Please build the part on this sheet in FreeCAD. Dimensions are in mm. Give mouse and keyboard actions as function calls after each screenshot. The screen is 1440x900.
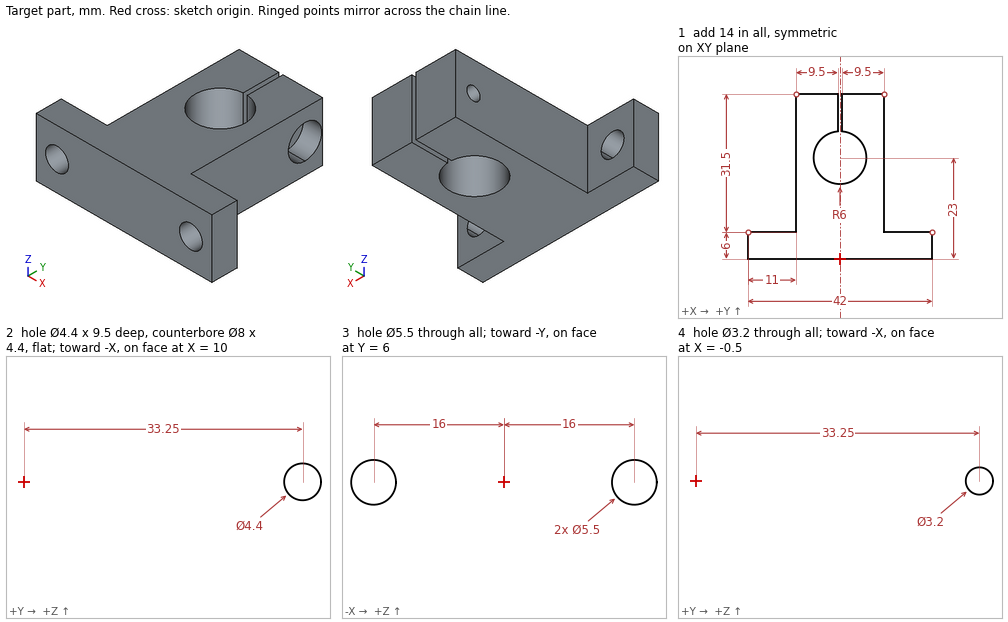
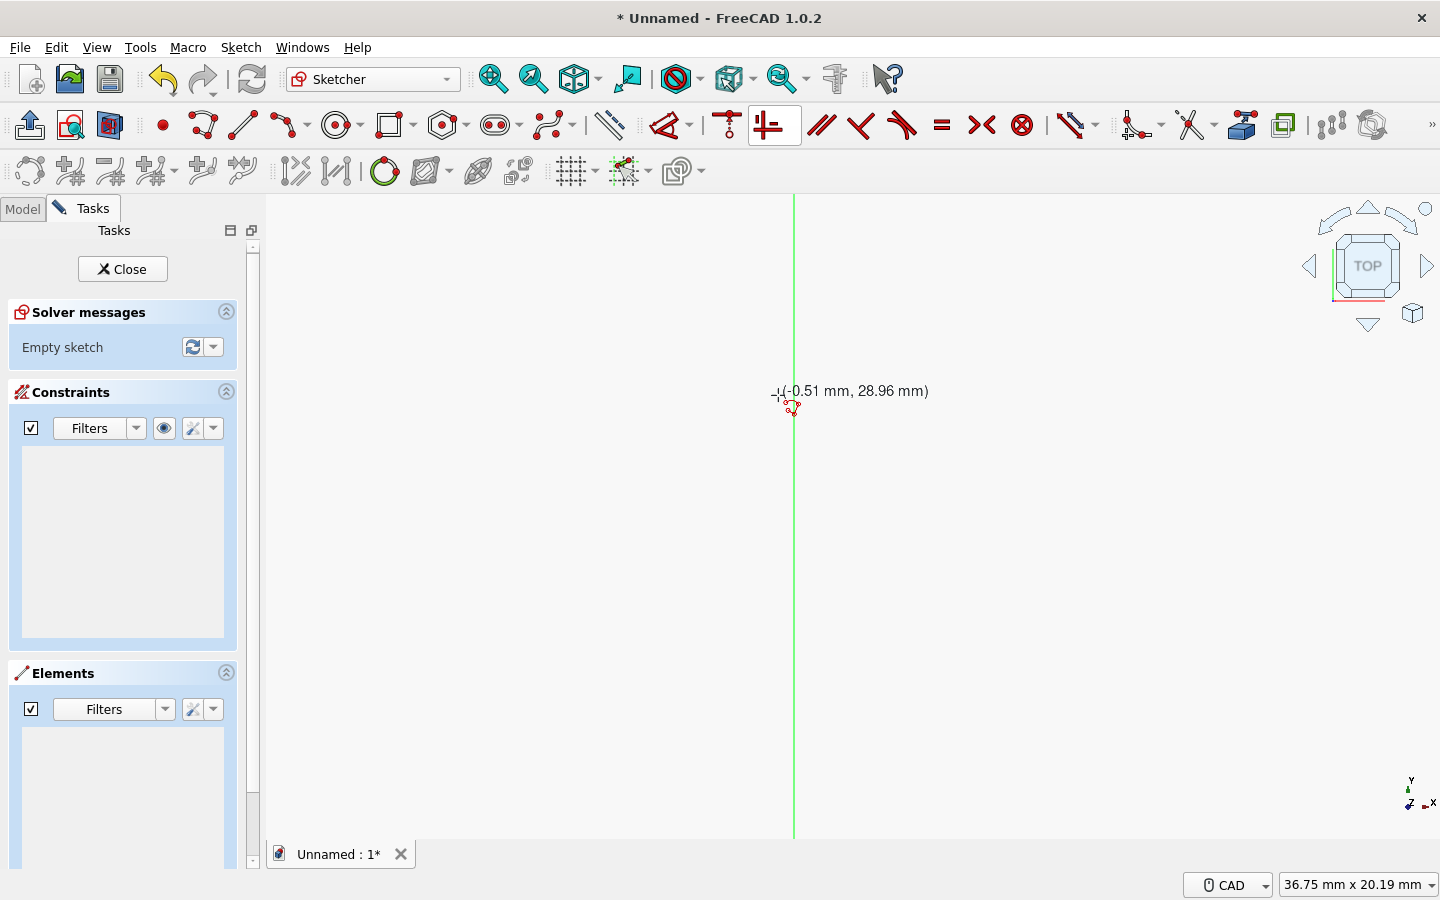
scroll(779, 397, down, 5)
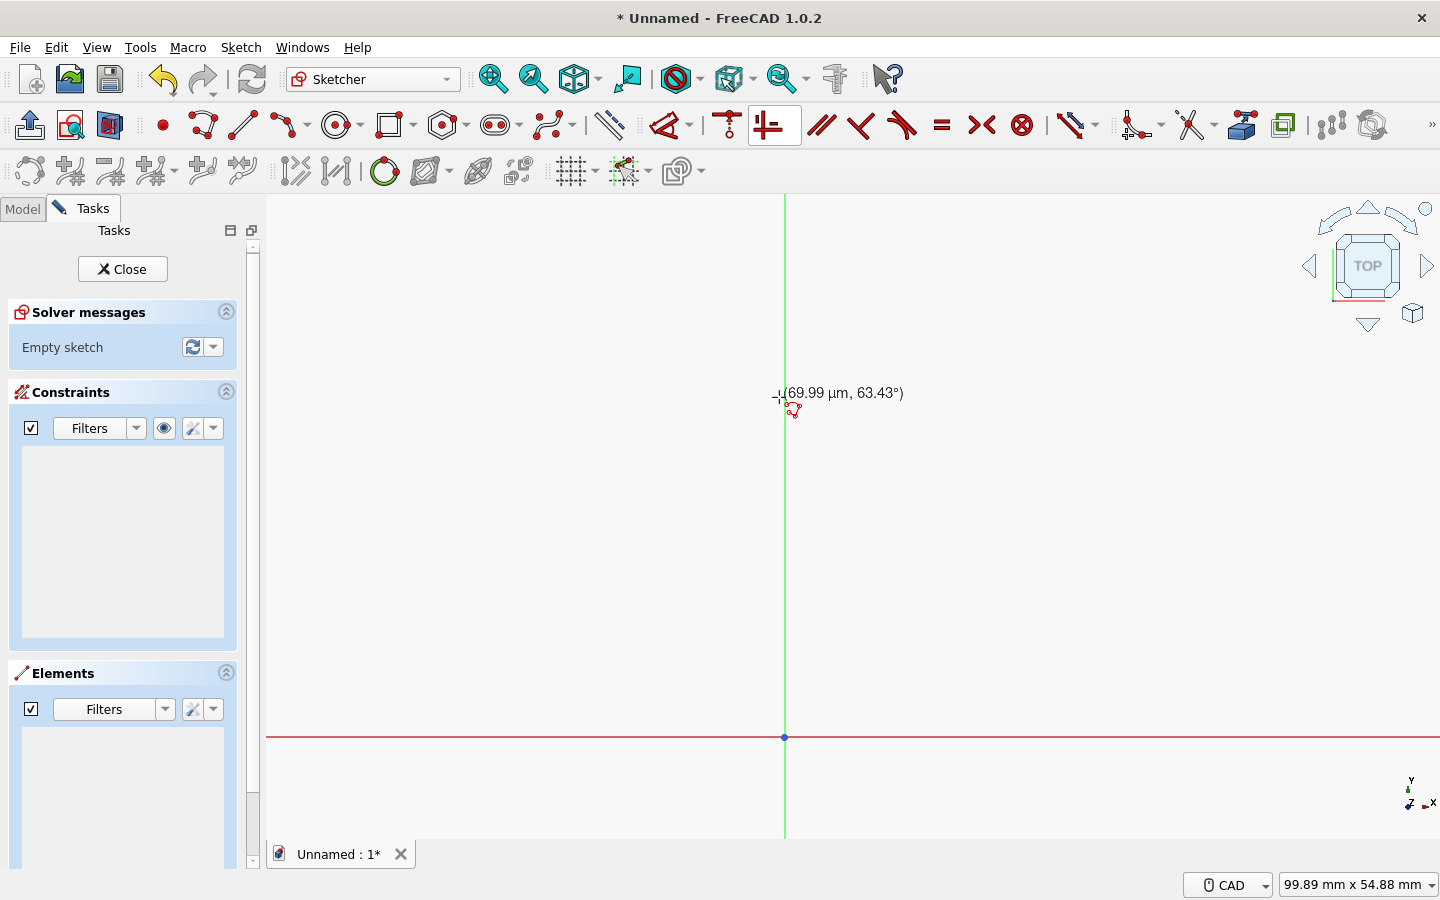
scroll(779, 296, up, 5)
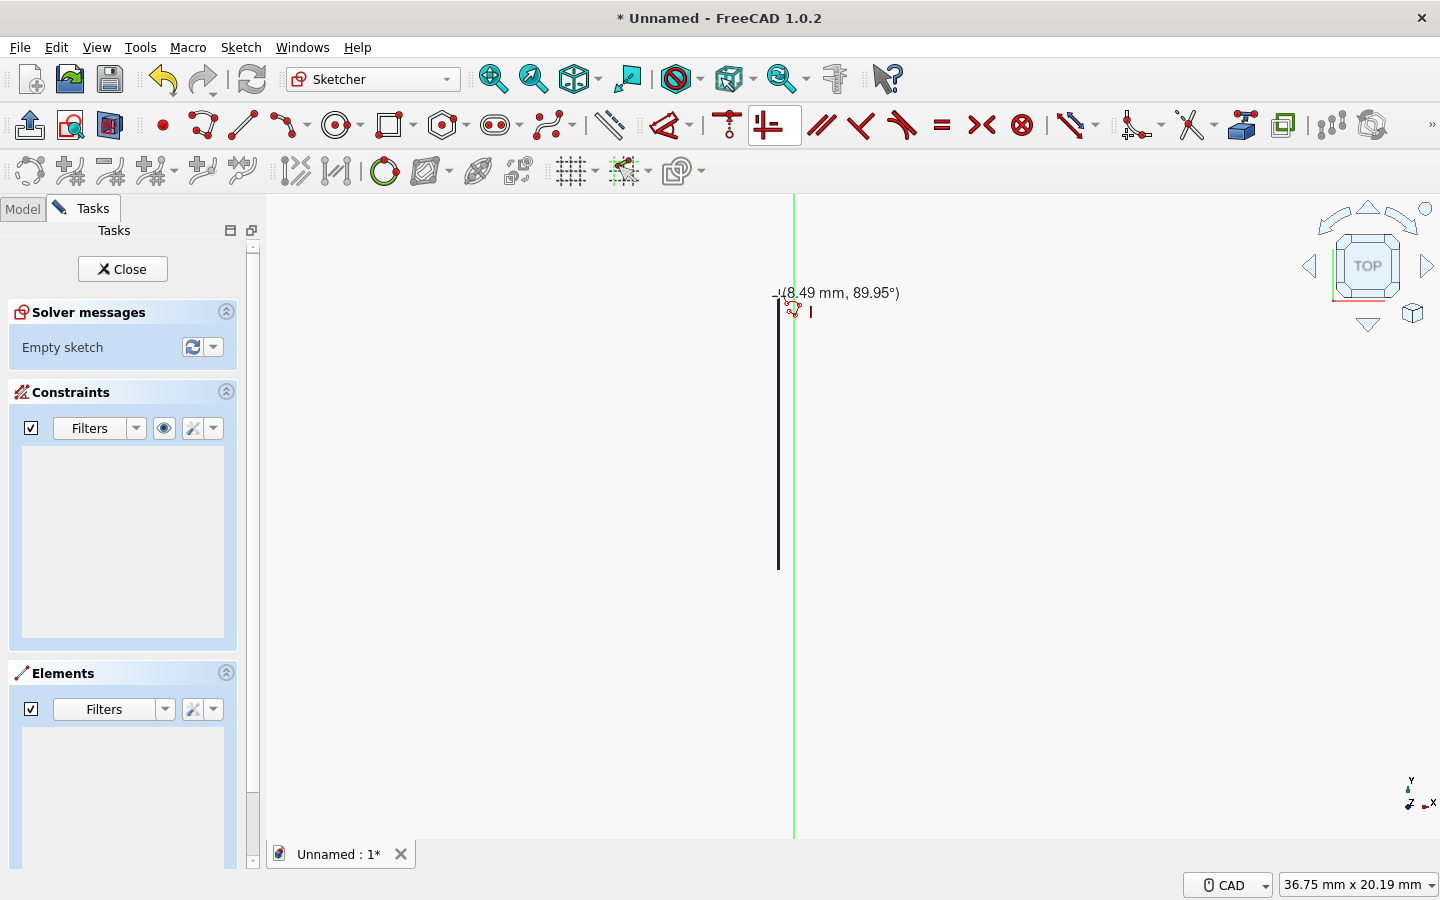
click(778, 297)
click(475, 297)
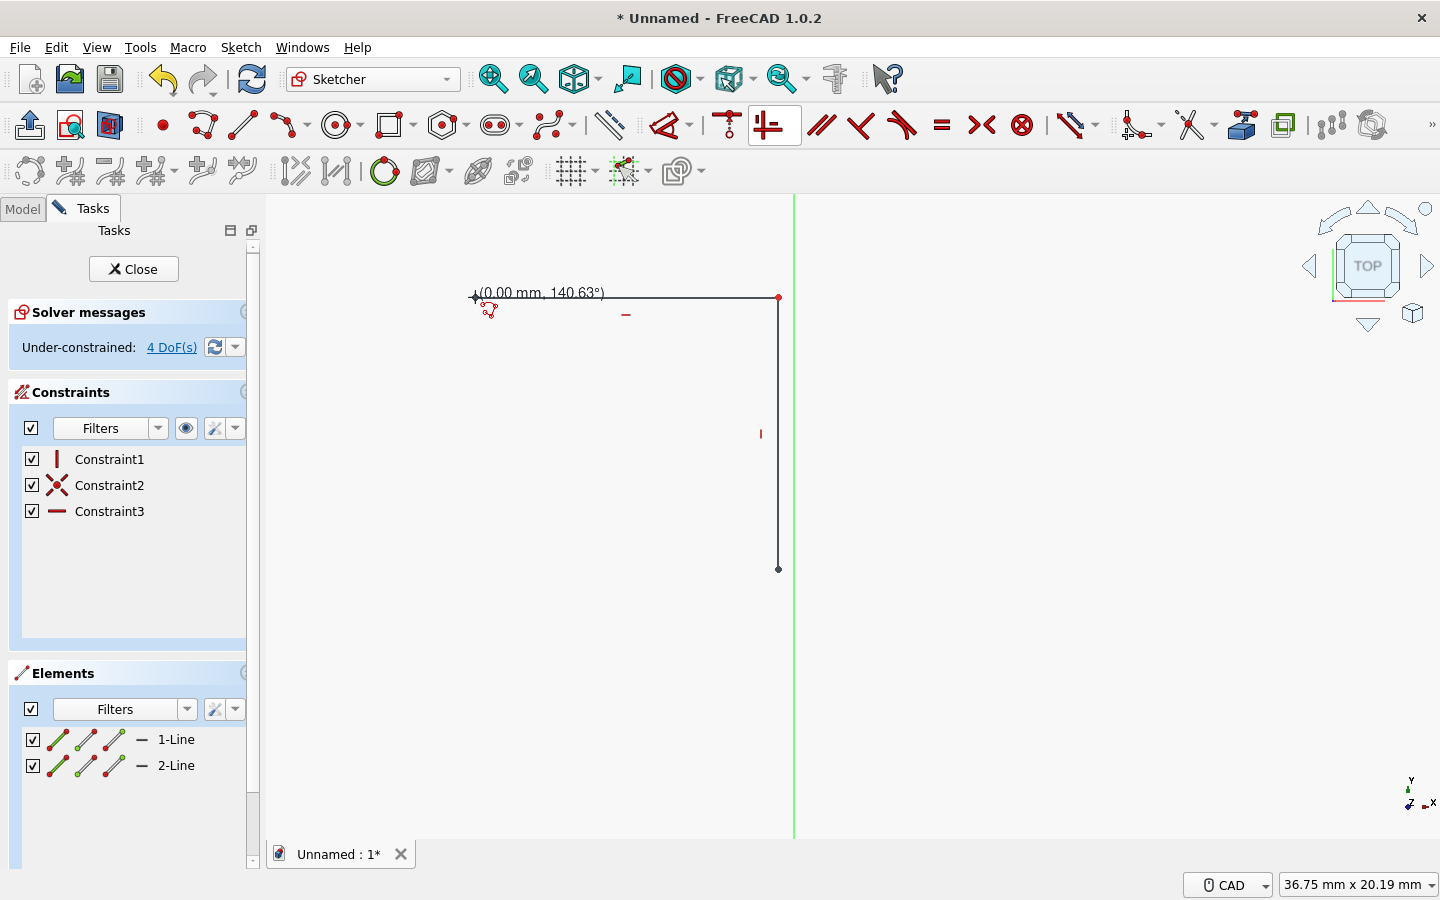
scroll(779, 296, down, 5)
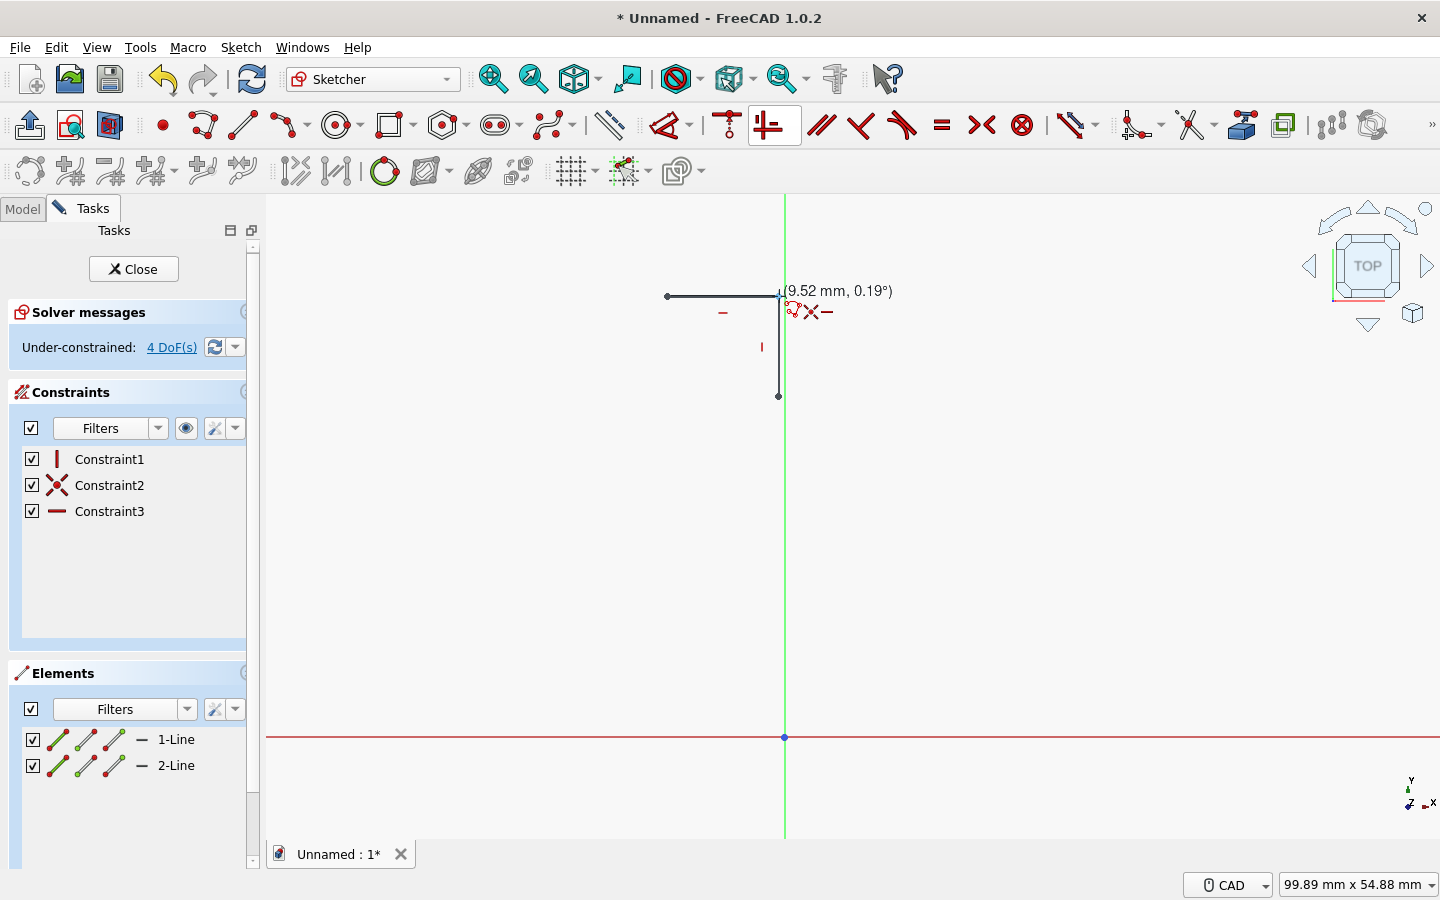
click(667, 667)
click(538, 667)
click(538, 737)
click(1032, 728)
click(1032, 667)
click(902, 667)
click(902, 296)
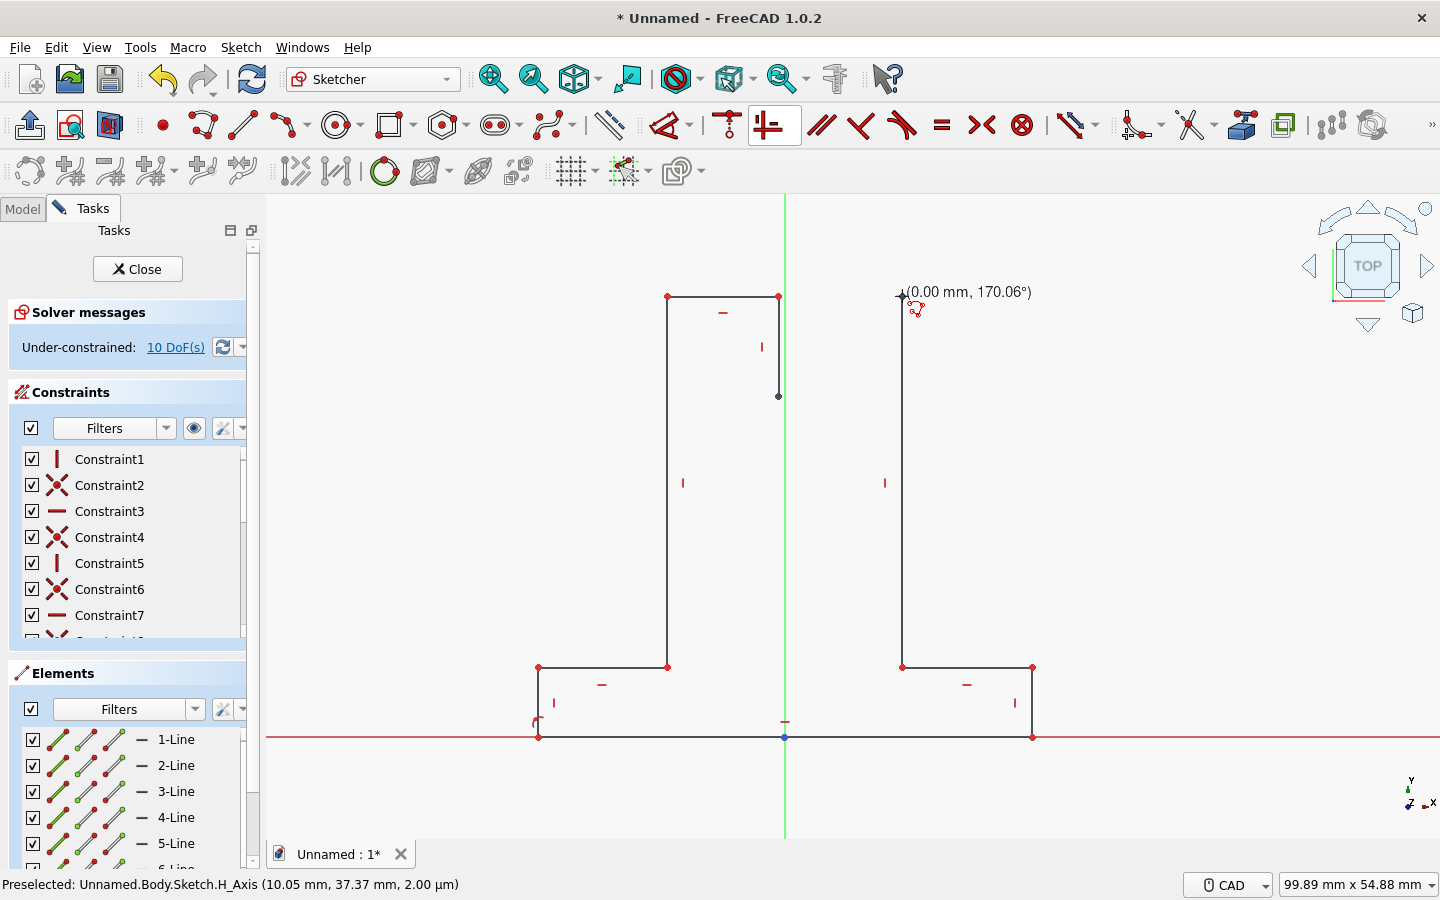
scroll(791, 296, up, 5)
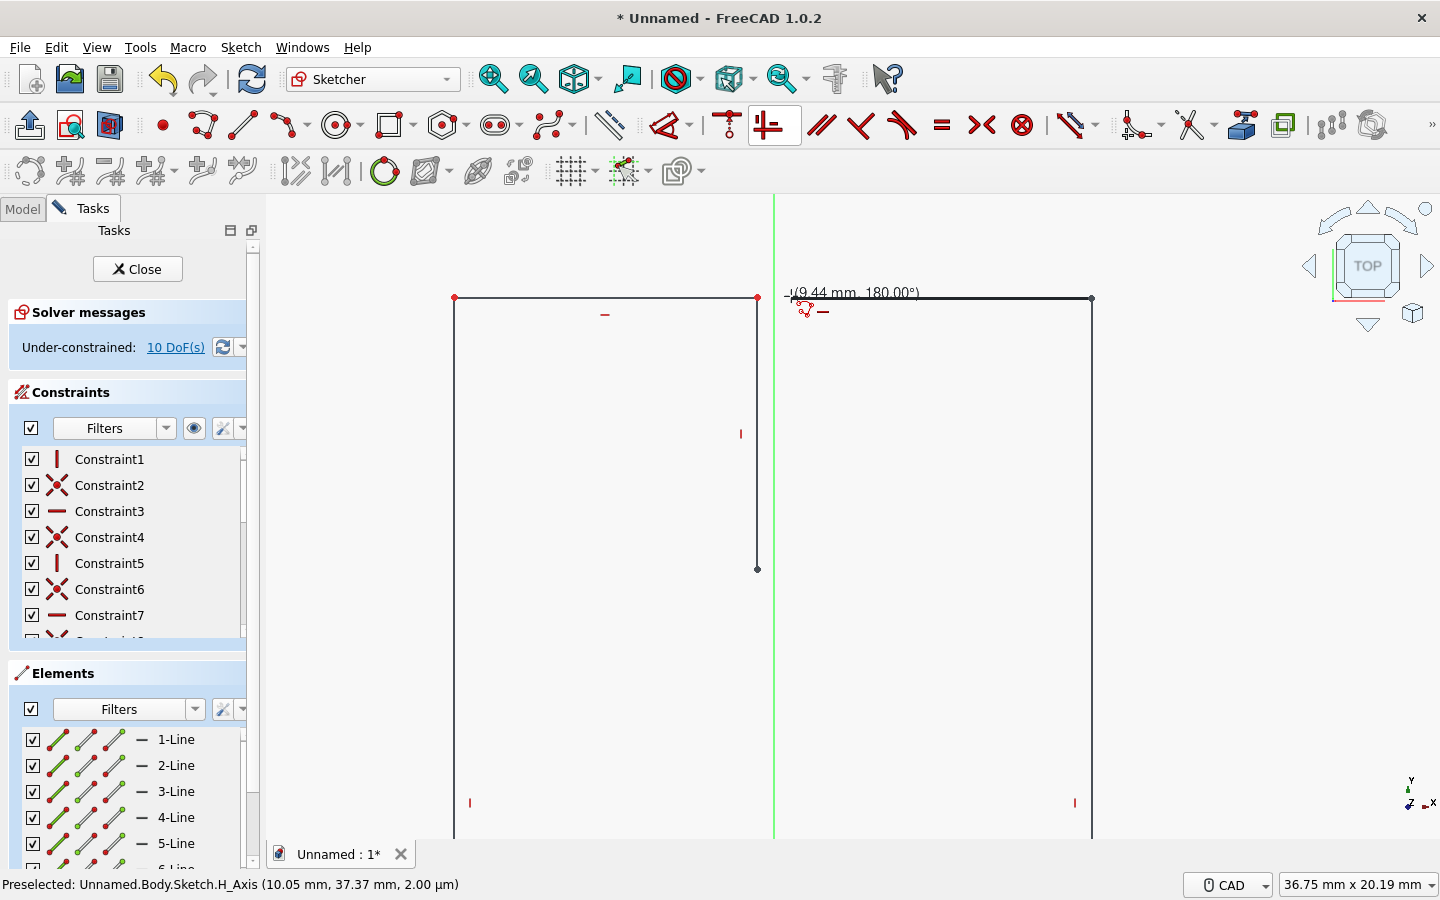
click(790, 296)
click(790, 569)
right_click(790, 569)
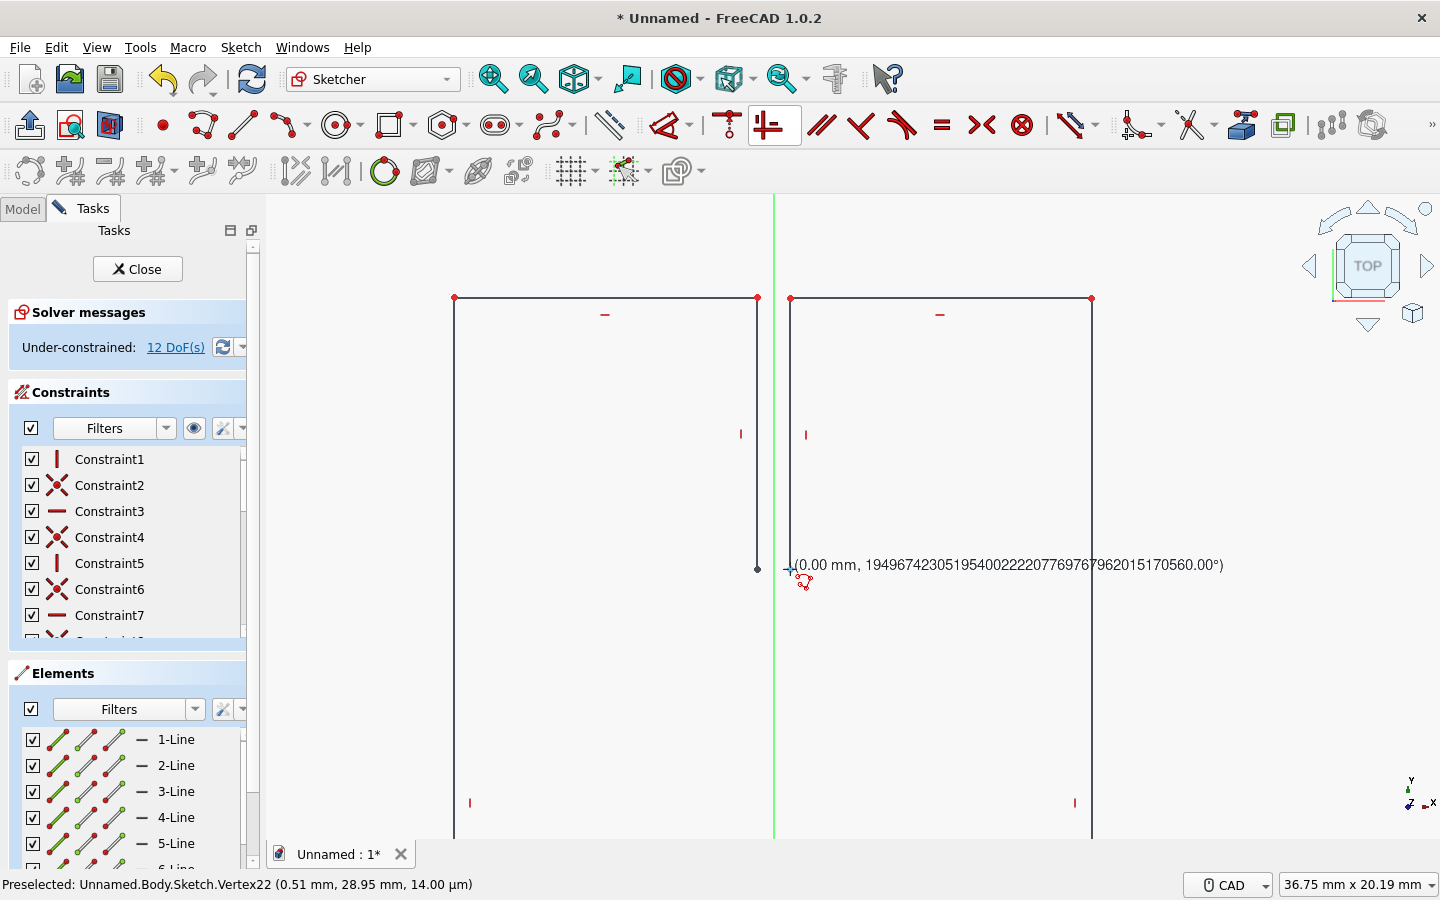
click(284, 126)